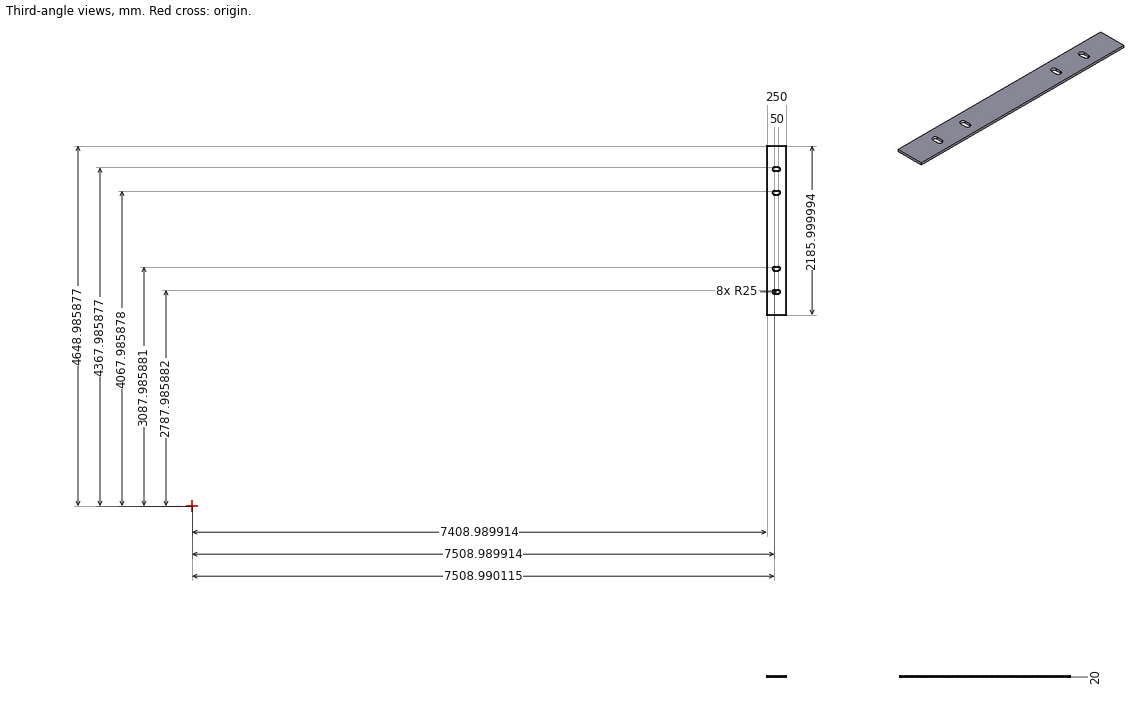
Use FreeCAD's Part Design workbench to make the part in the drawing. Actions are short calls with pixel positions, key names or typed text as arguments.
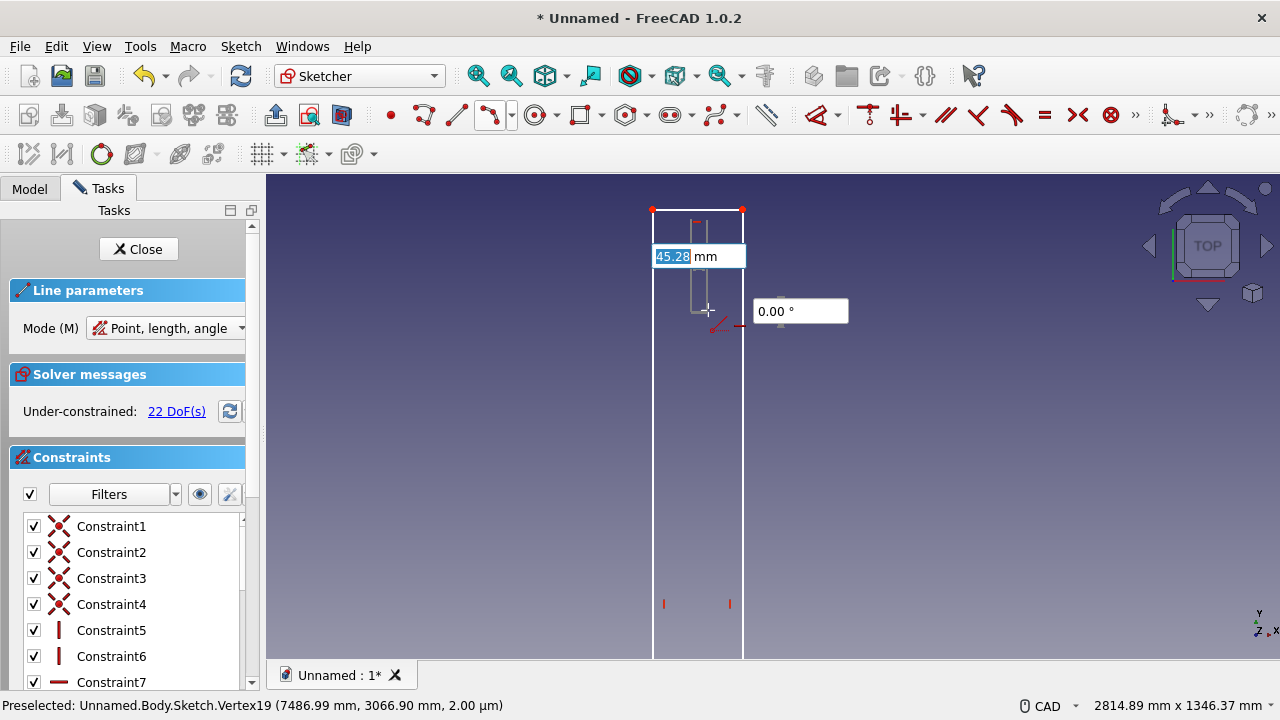
click(708, 310)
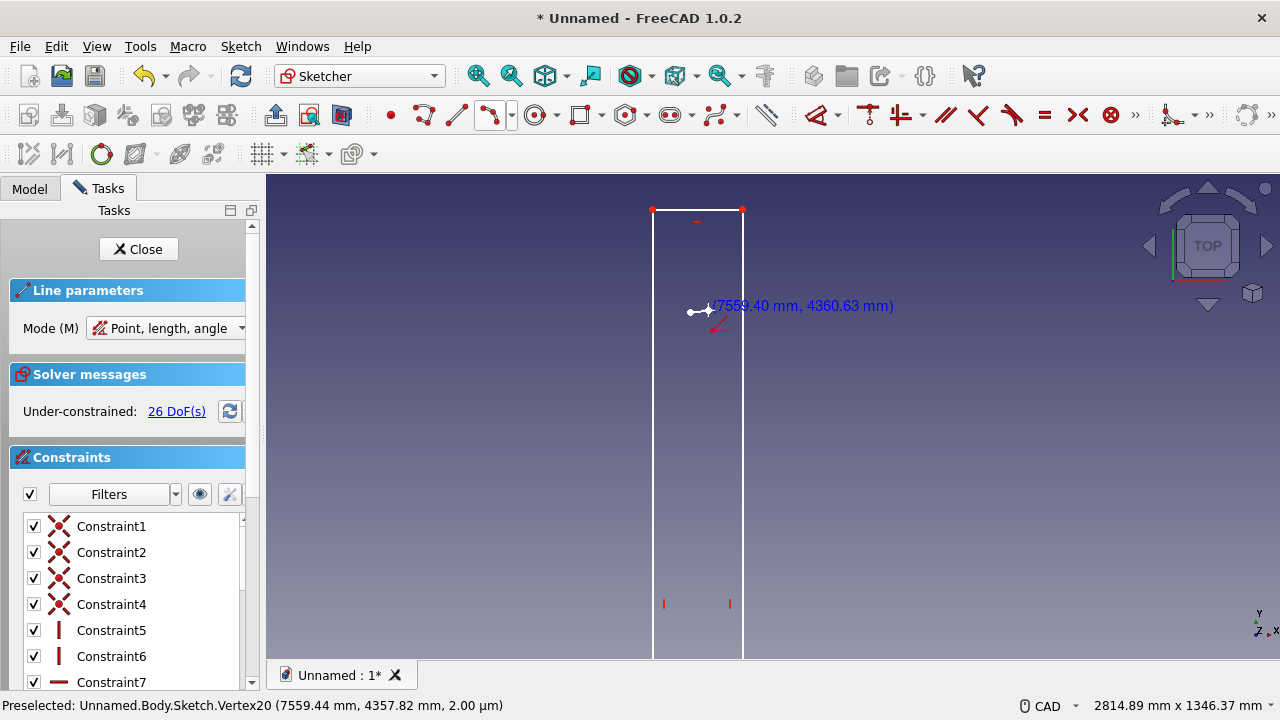
click(708, 326)
click(690, 326)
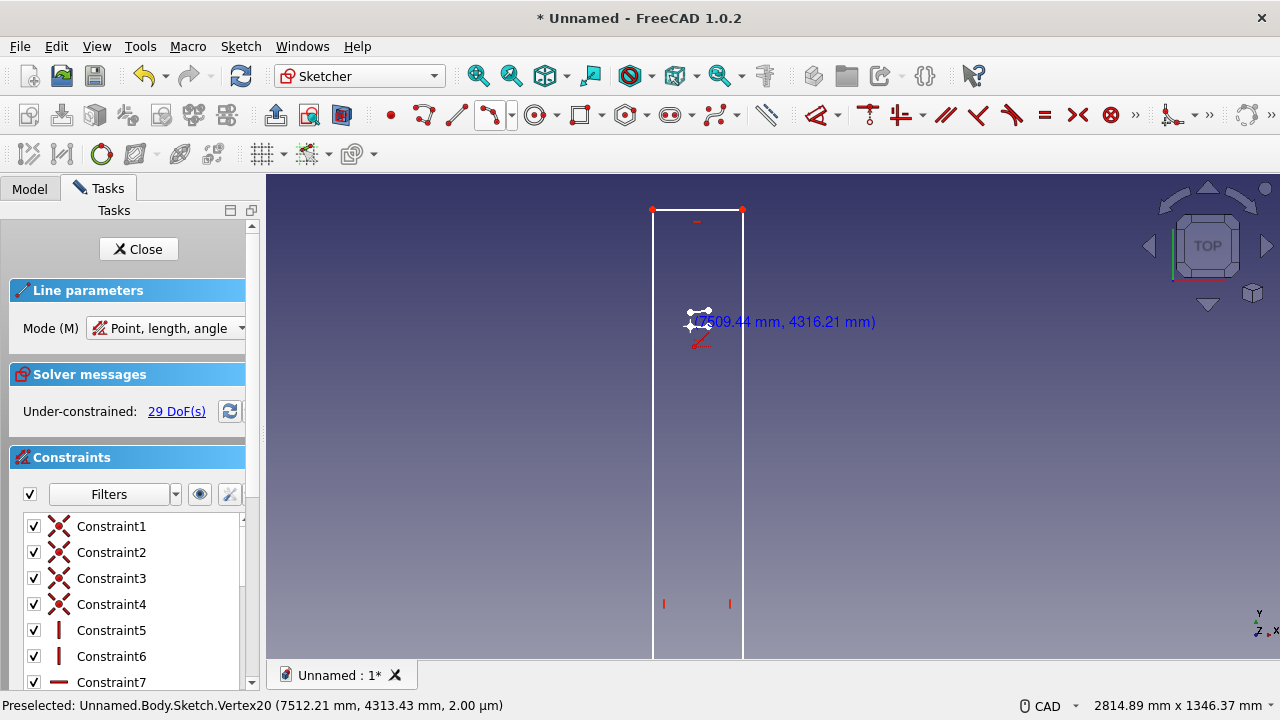
key(g)
key(3)
key(a)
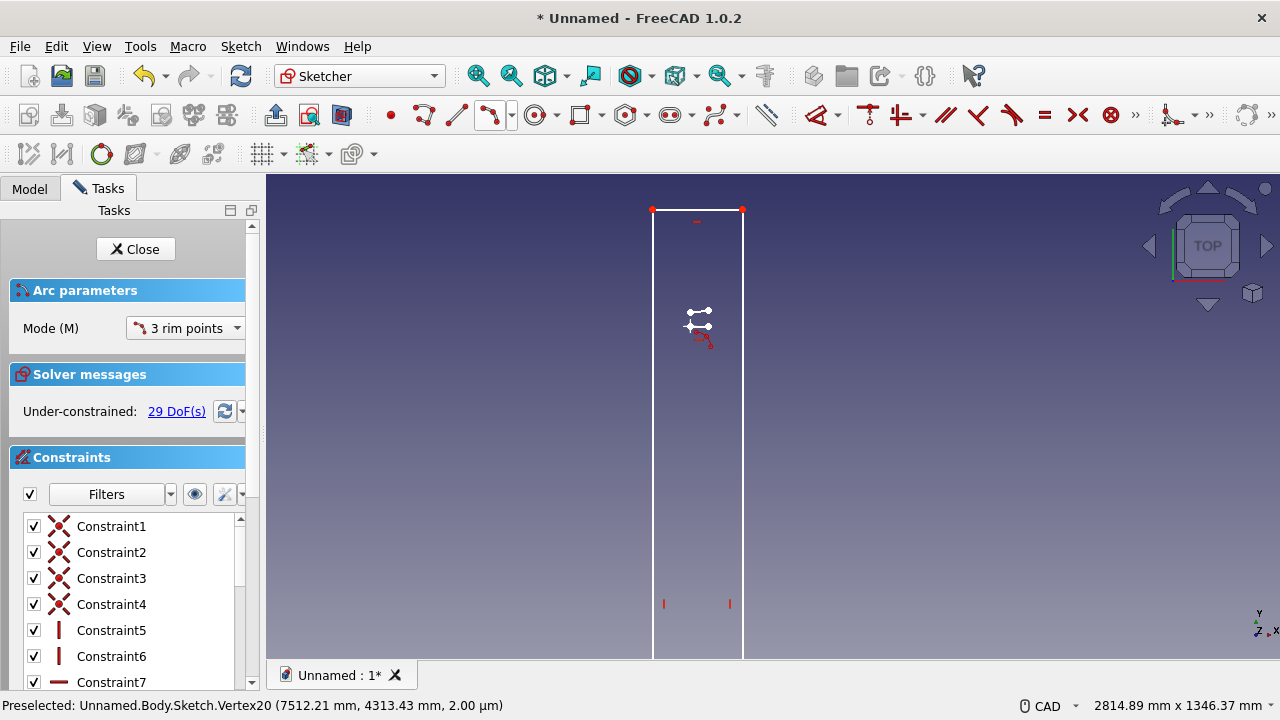
scroll(708, 308, up, 3)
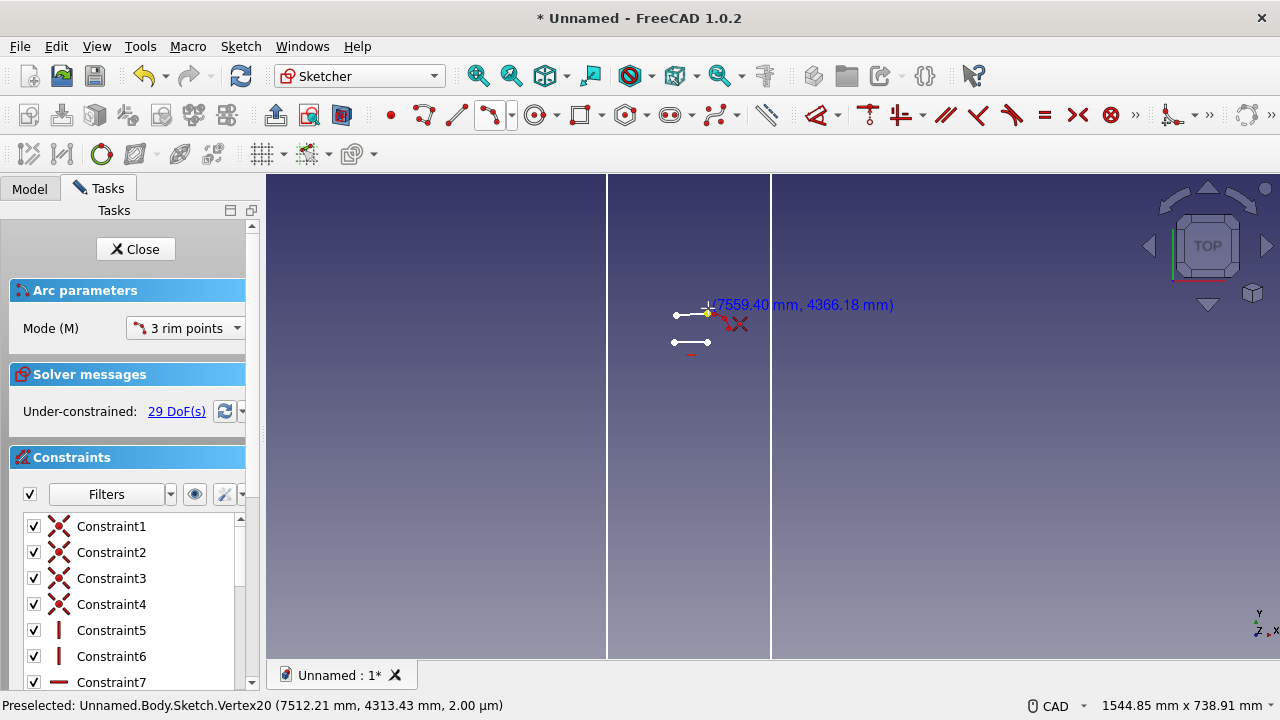
click(708, 313)
click(708, 342)
click(724, 325)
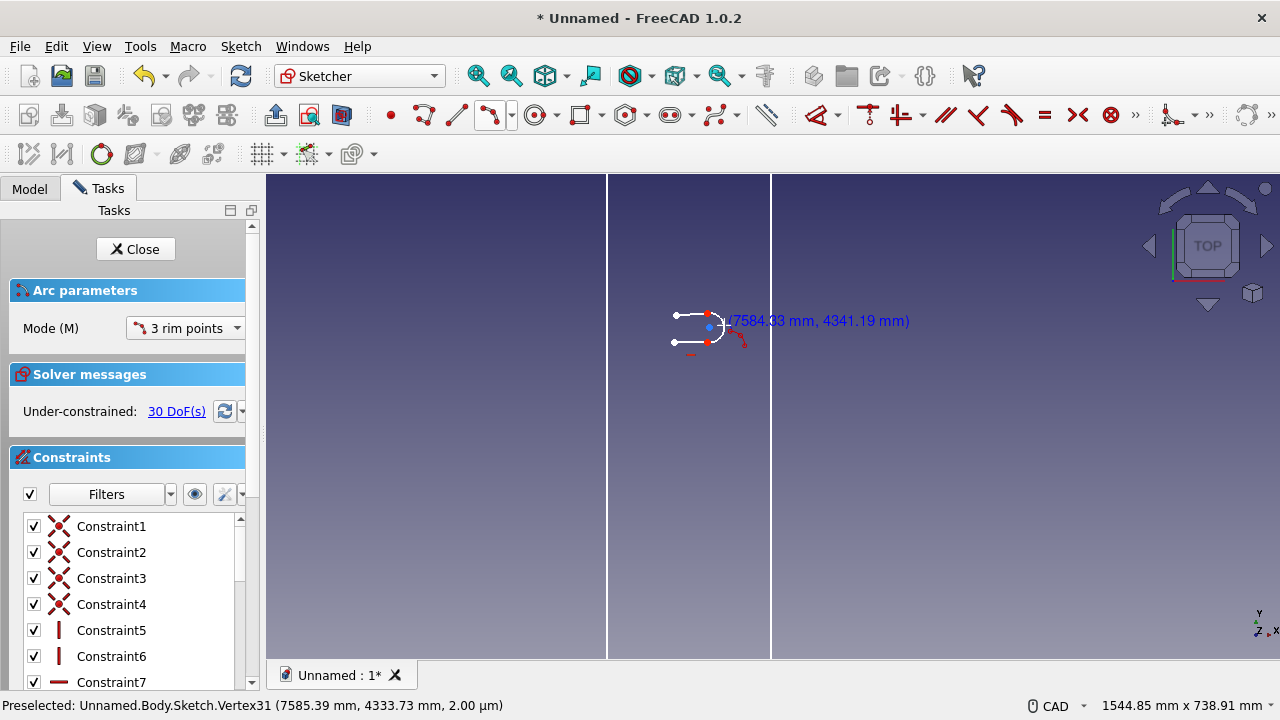
click(675, 342)
click(677, 315)
click(658, 325)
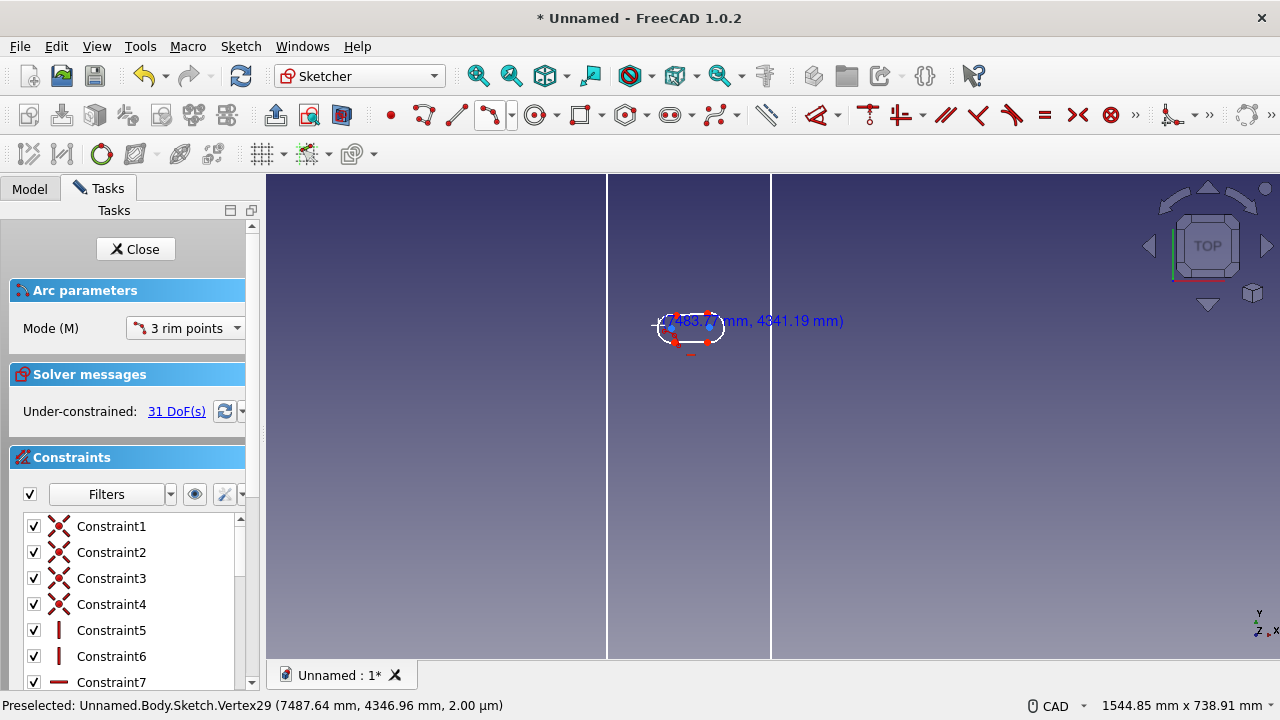
click(457, 116)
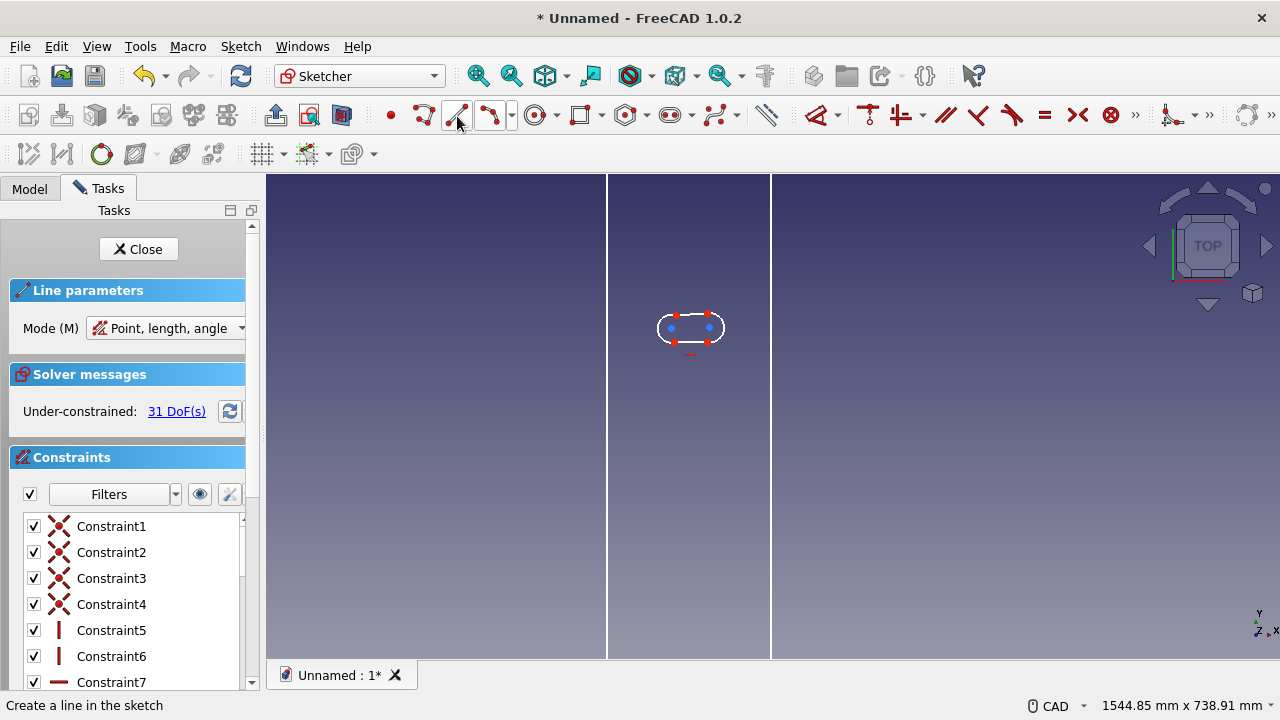
scroll(708, 309, down, 8)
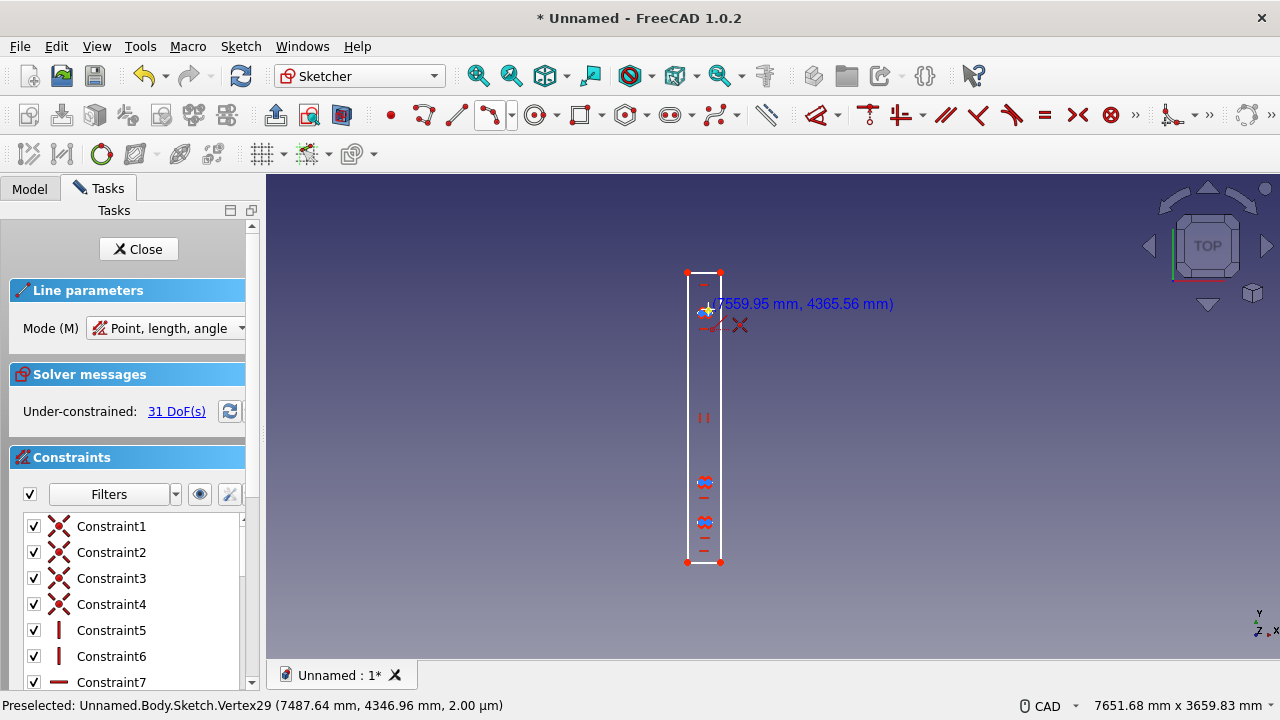
click(702, 349)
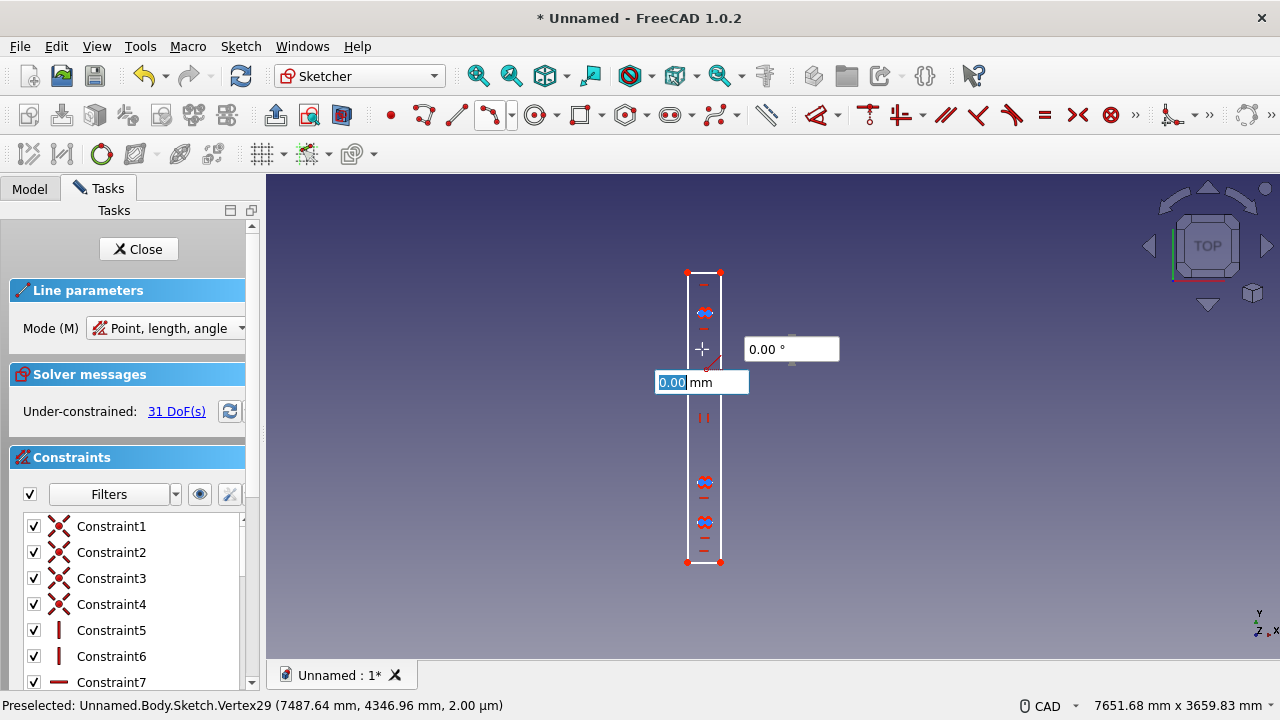
scroll(708, 349, up, 5)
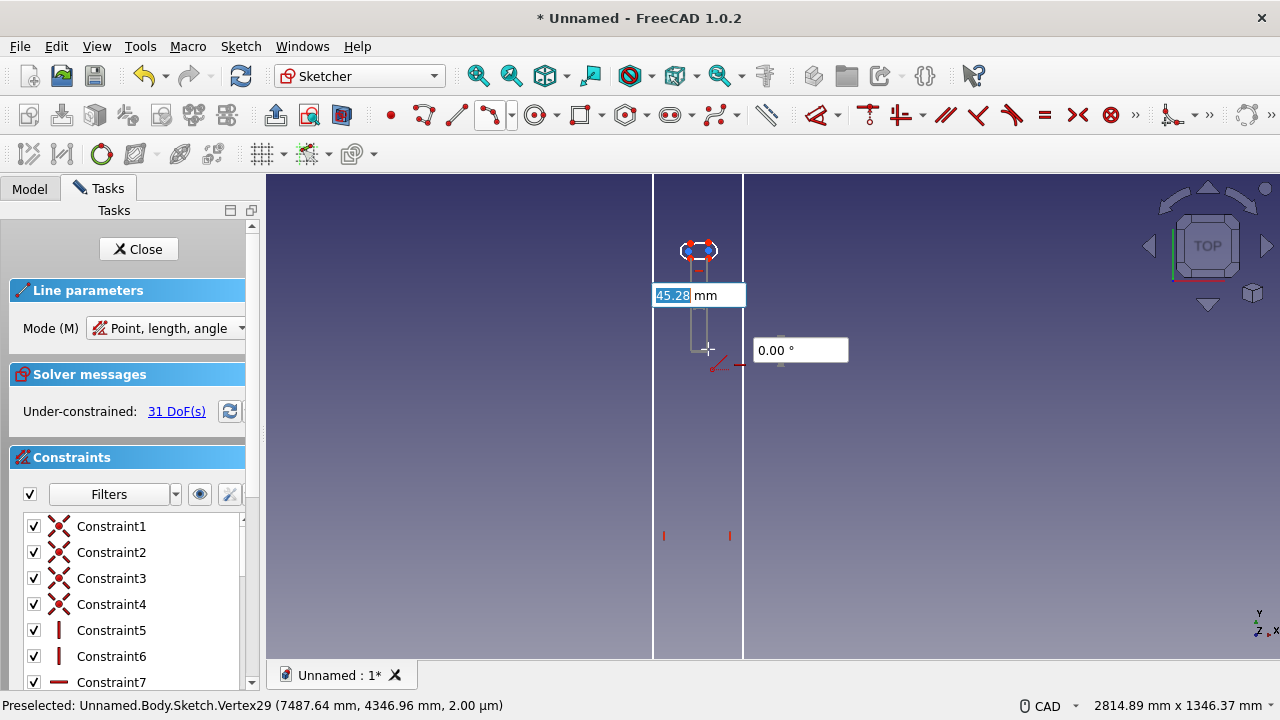
click(708, 348)